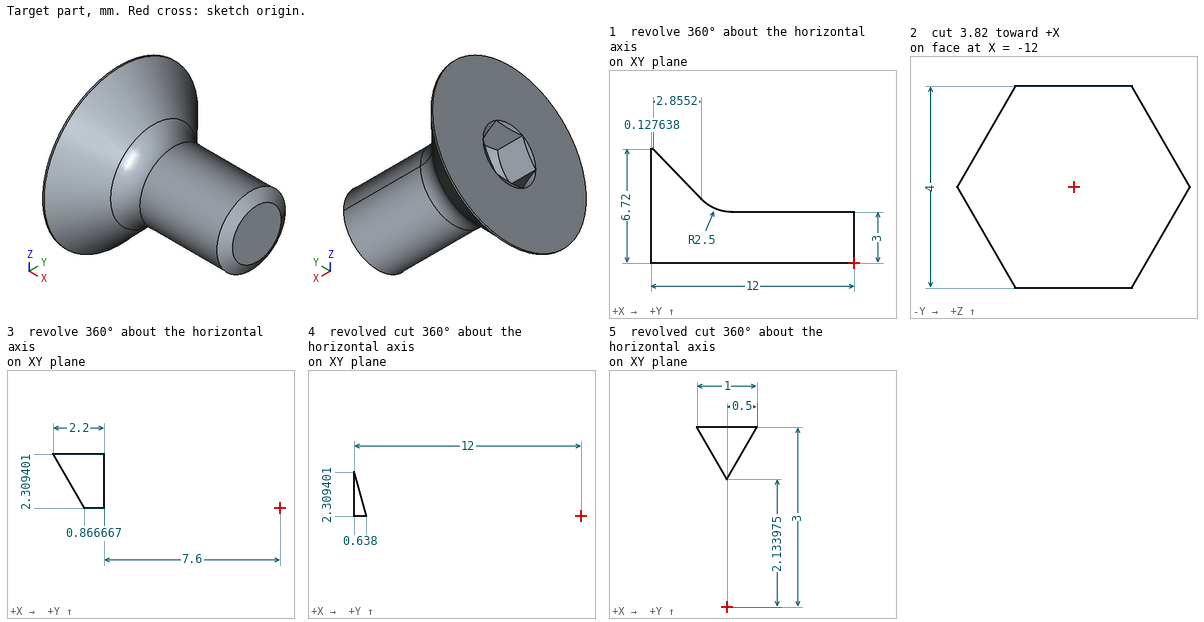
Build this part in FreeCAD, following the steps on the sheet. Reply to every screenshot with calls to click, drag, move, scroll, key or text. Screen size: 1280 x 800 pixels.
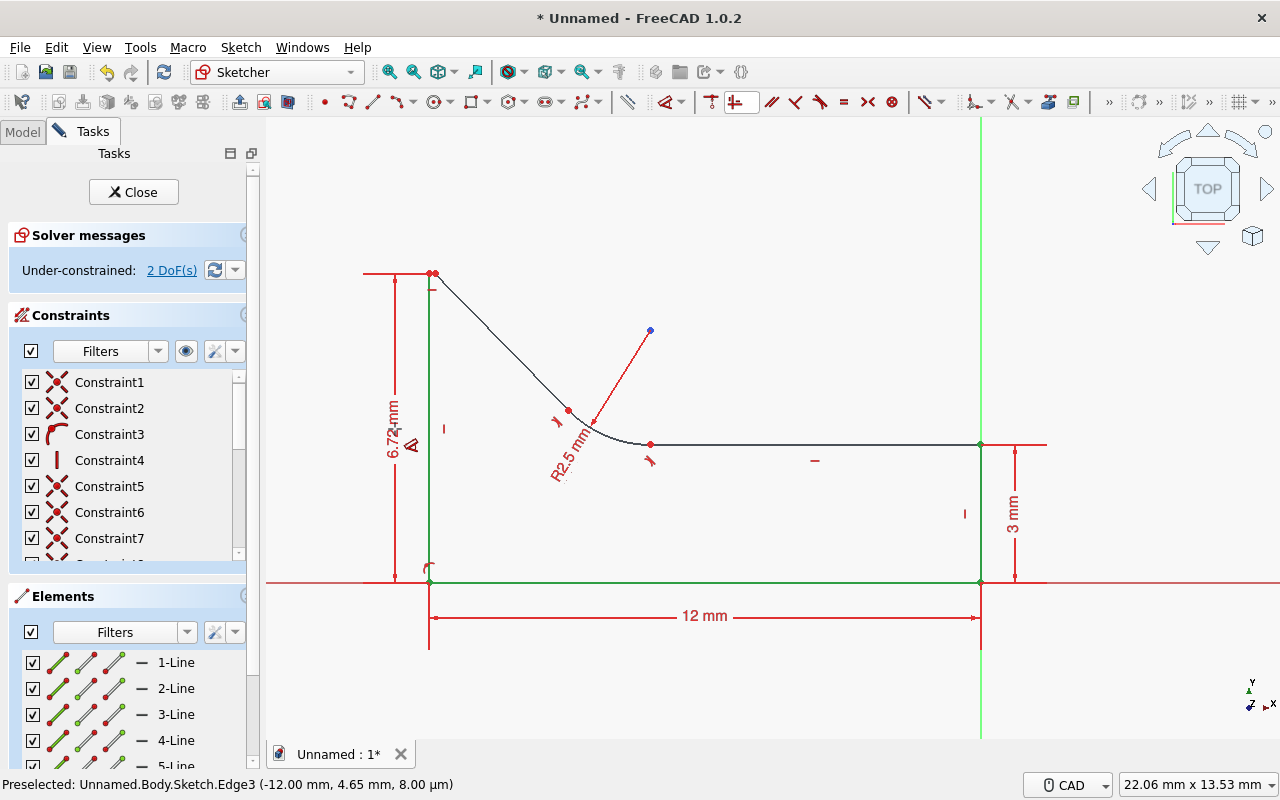
click(529, 369)
click(502, 240)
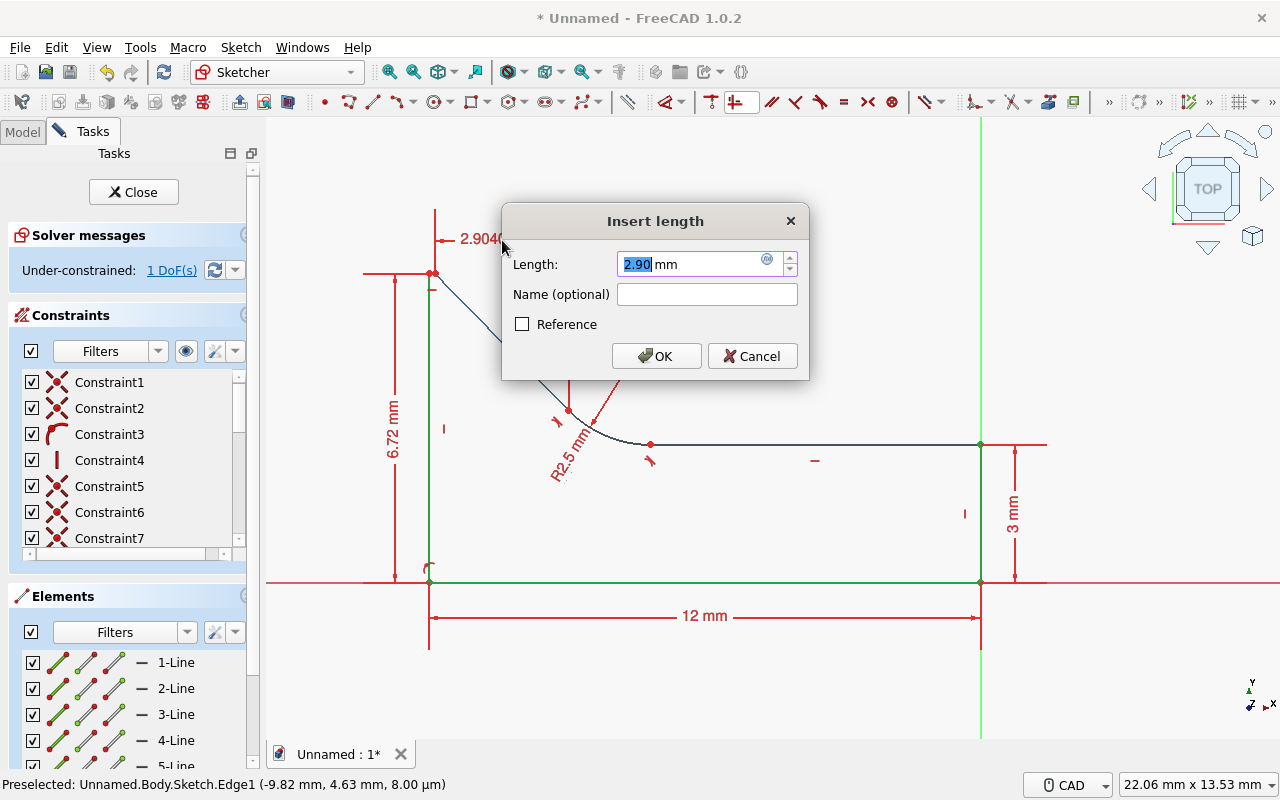
text(2.8552)
key(Return)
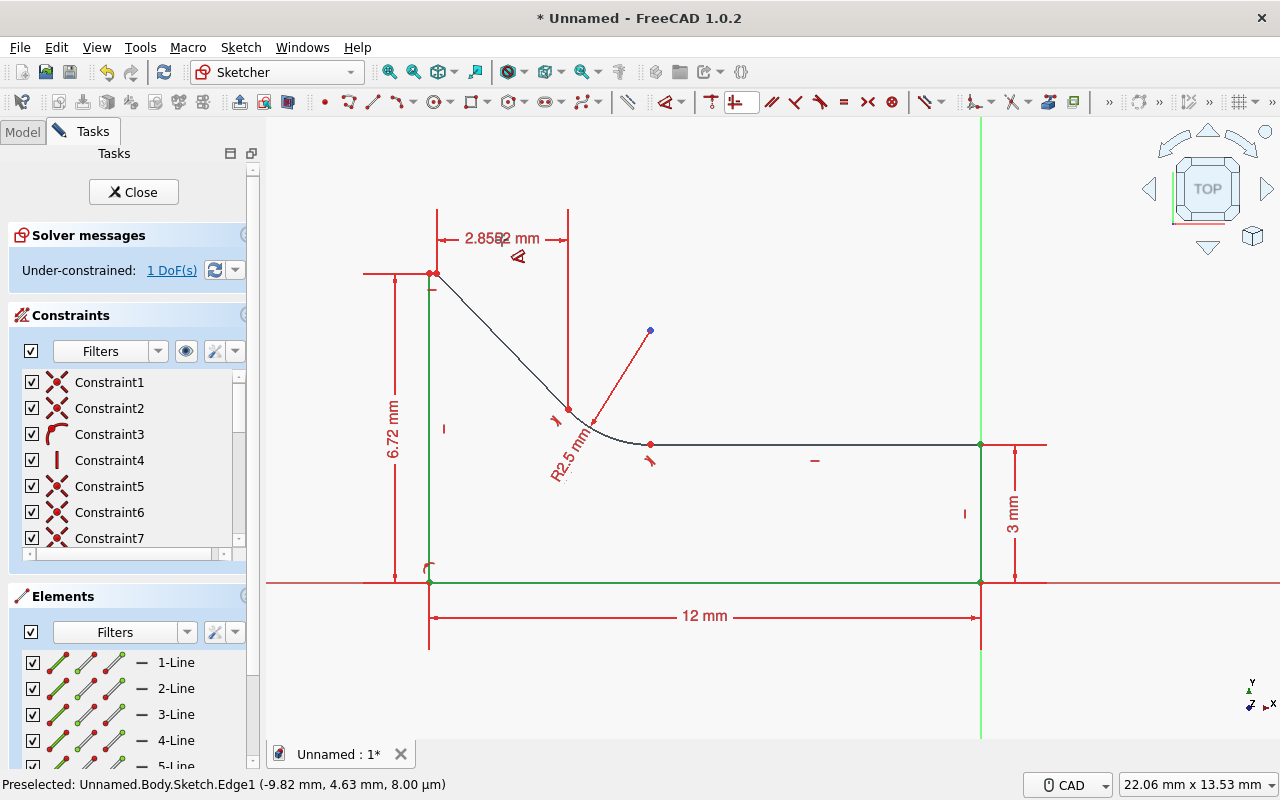
scroll(433, 274, up, 10)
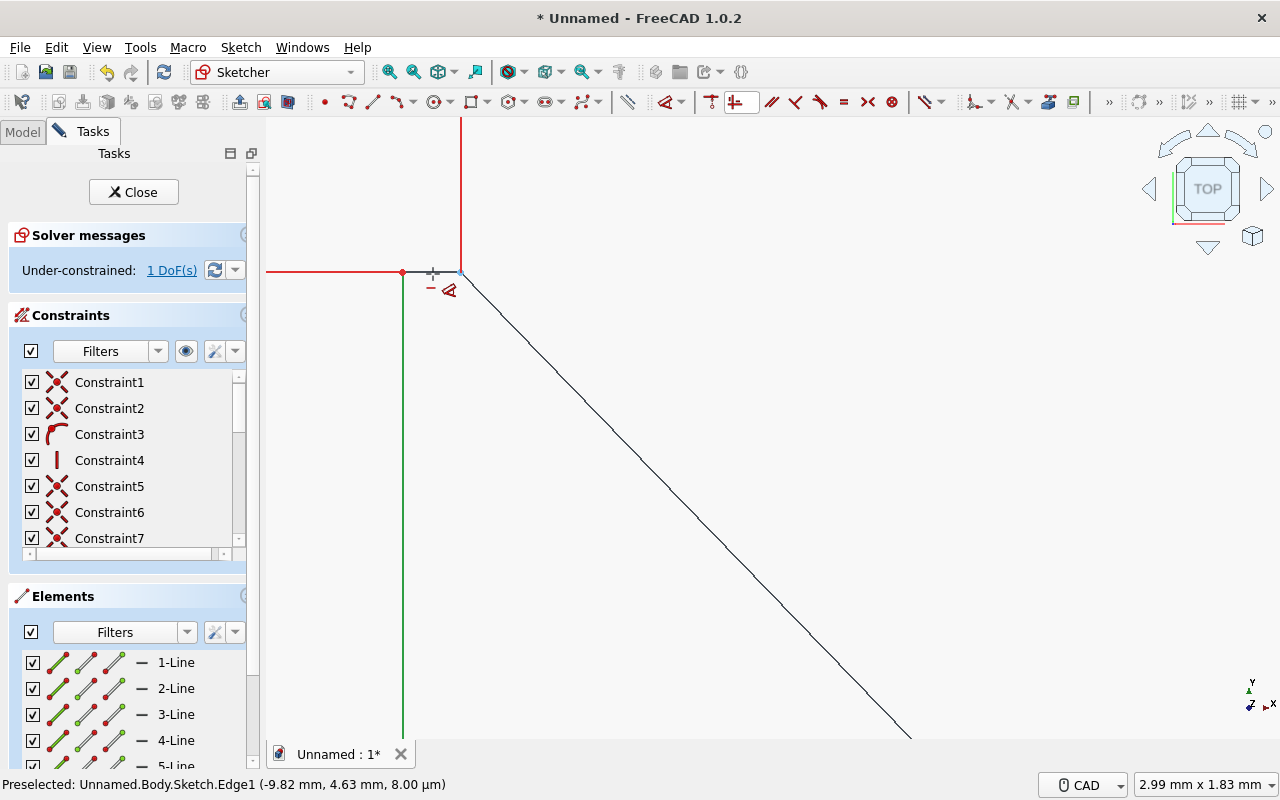
click(432, 272)
click(432, 238)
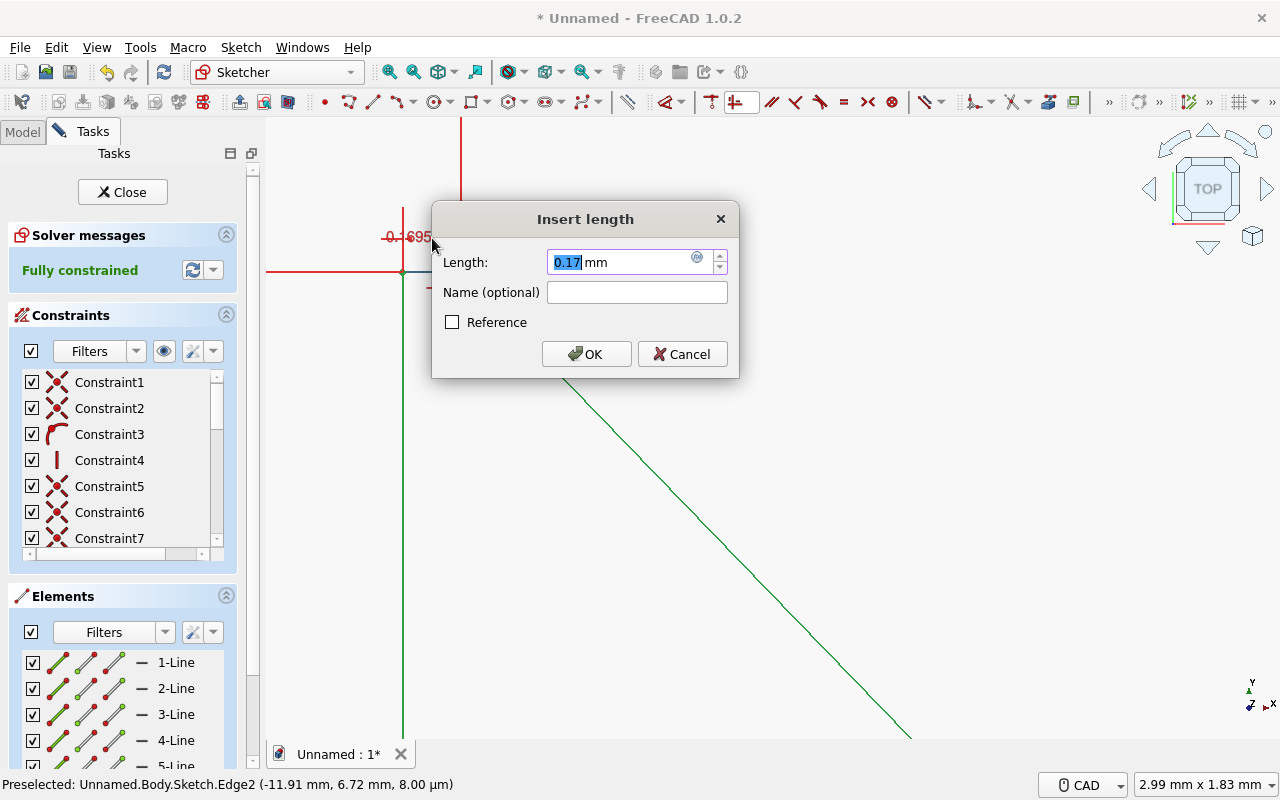
text(0.127638)
key(Return)
key(Escape)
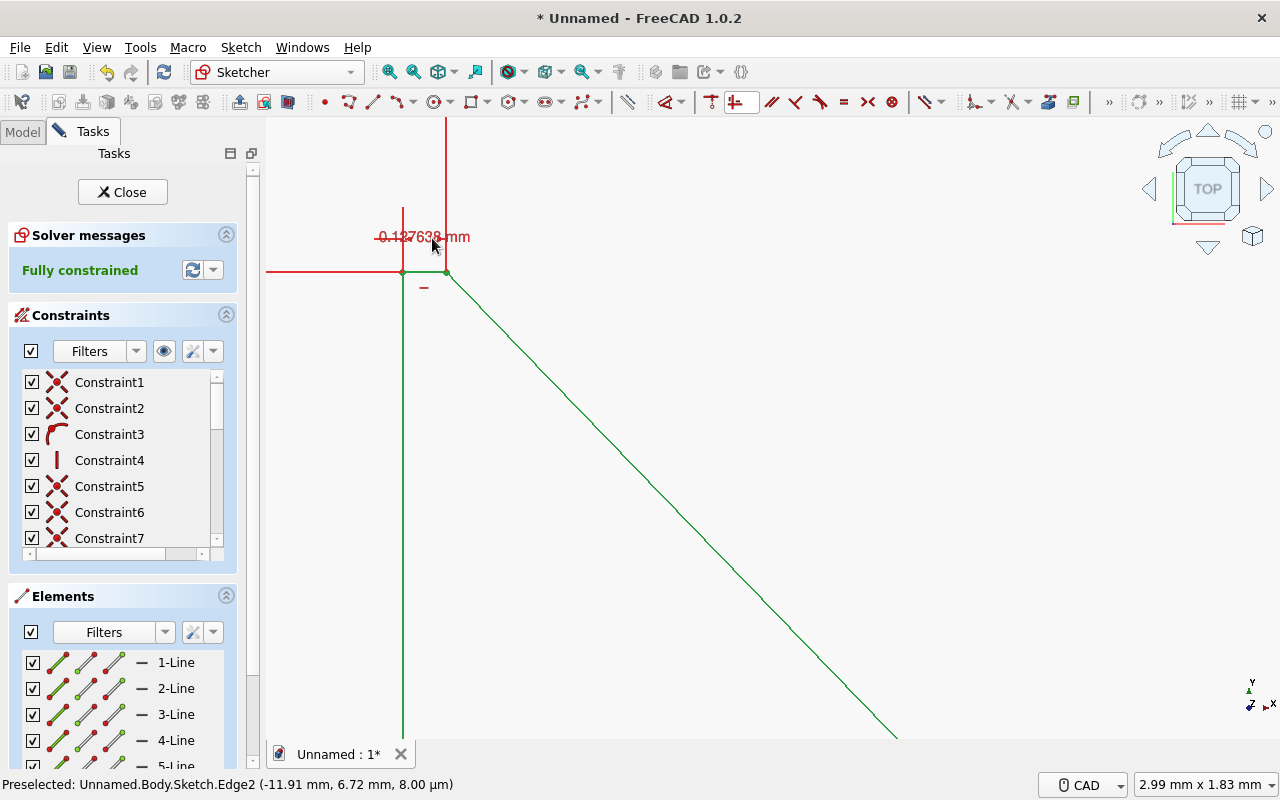
click(123, 192)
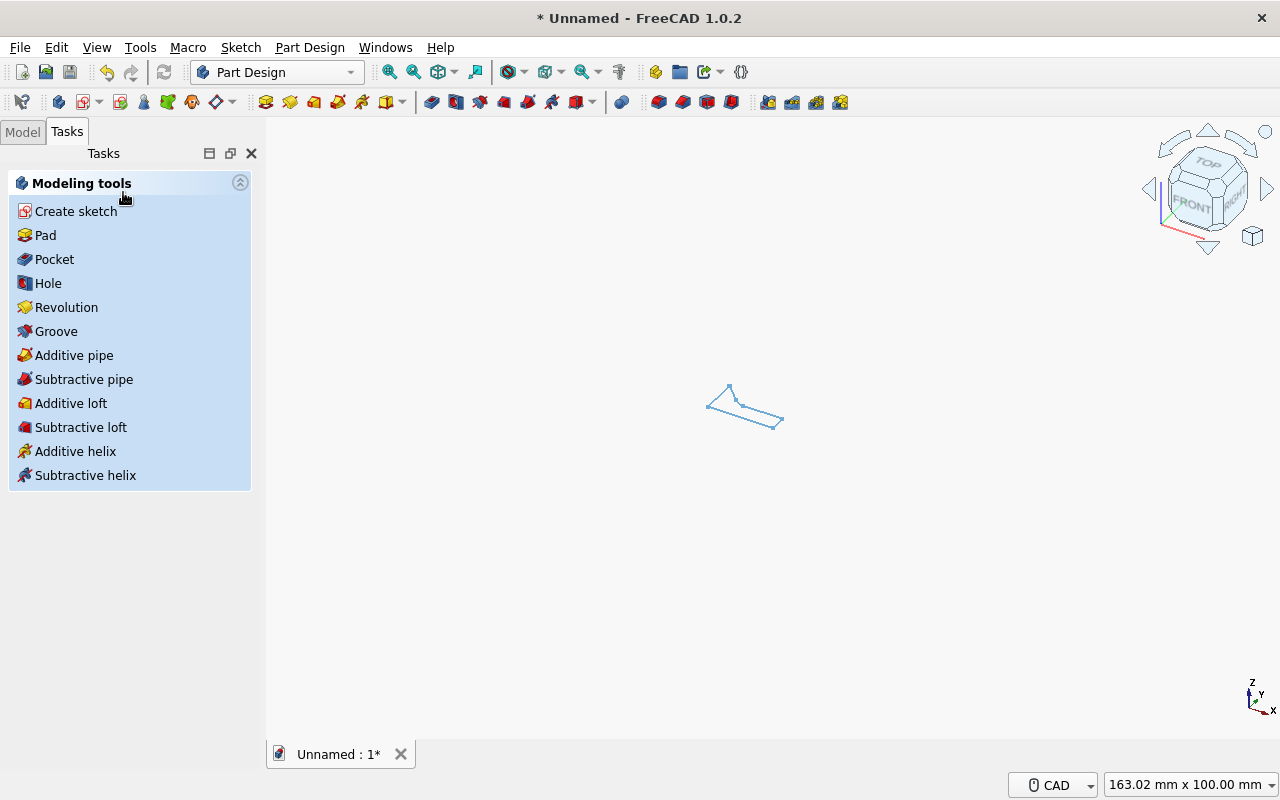
click(290, 102)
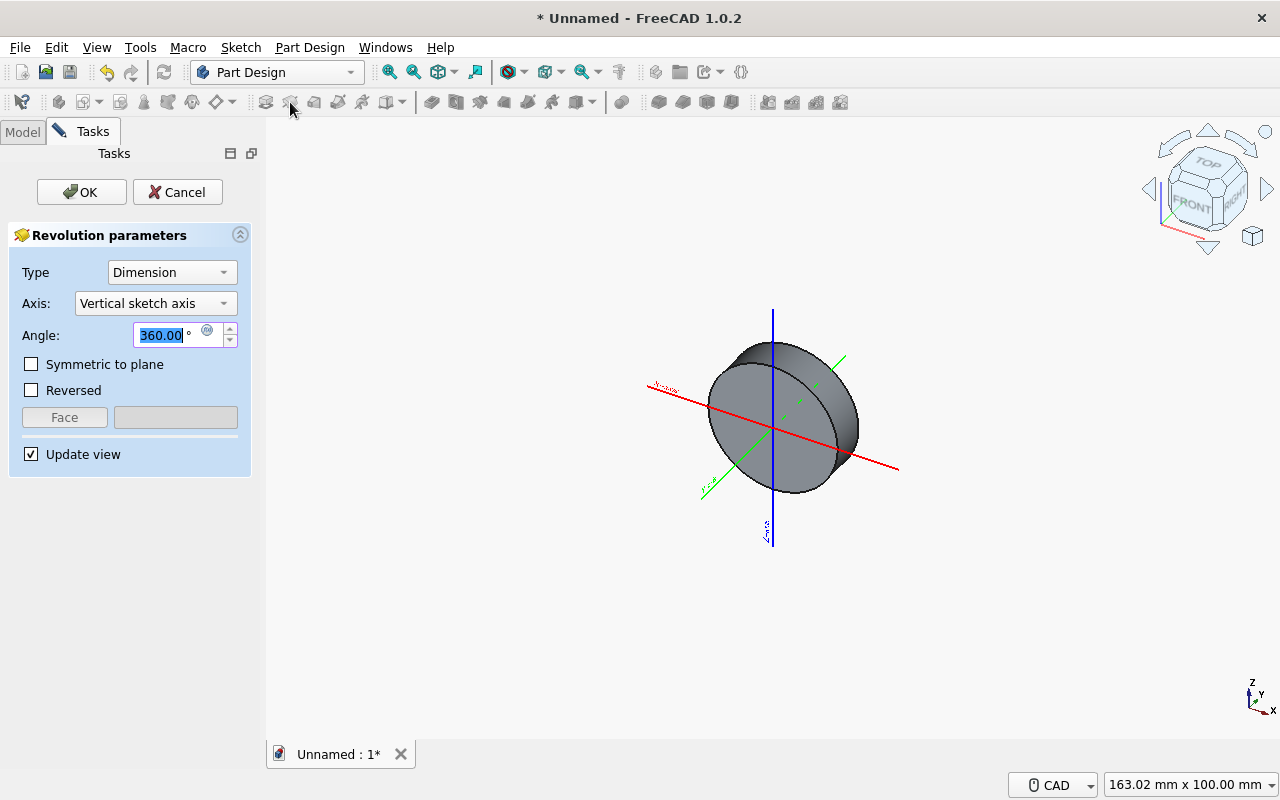
click(156, 304)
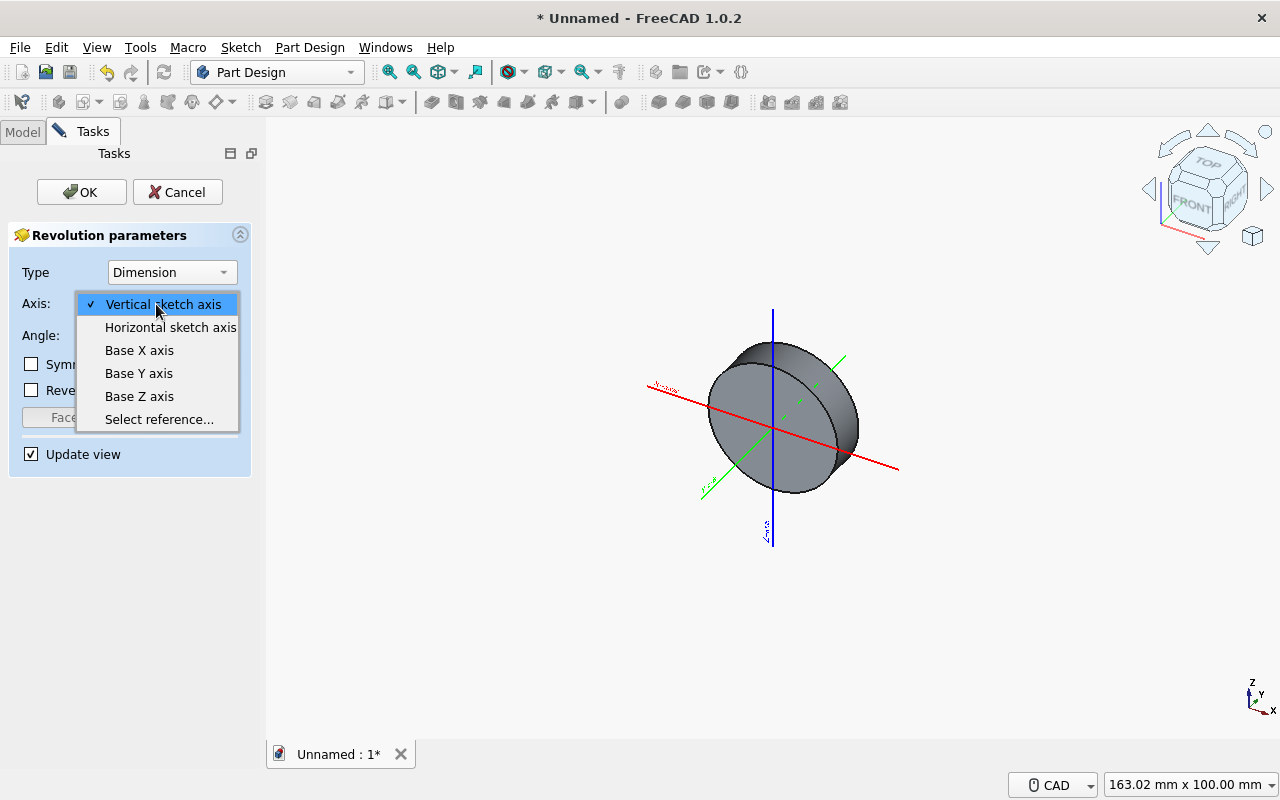
click(156, 328)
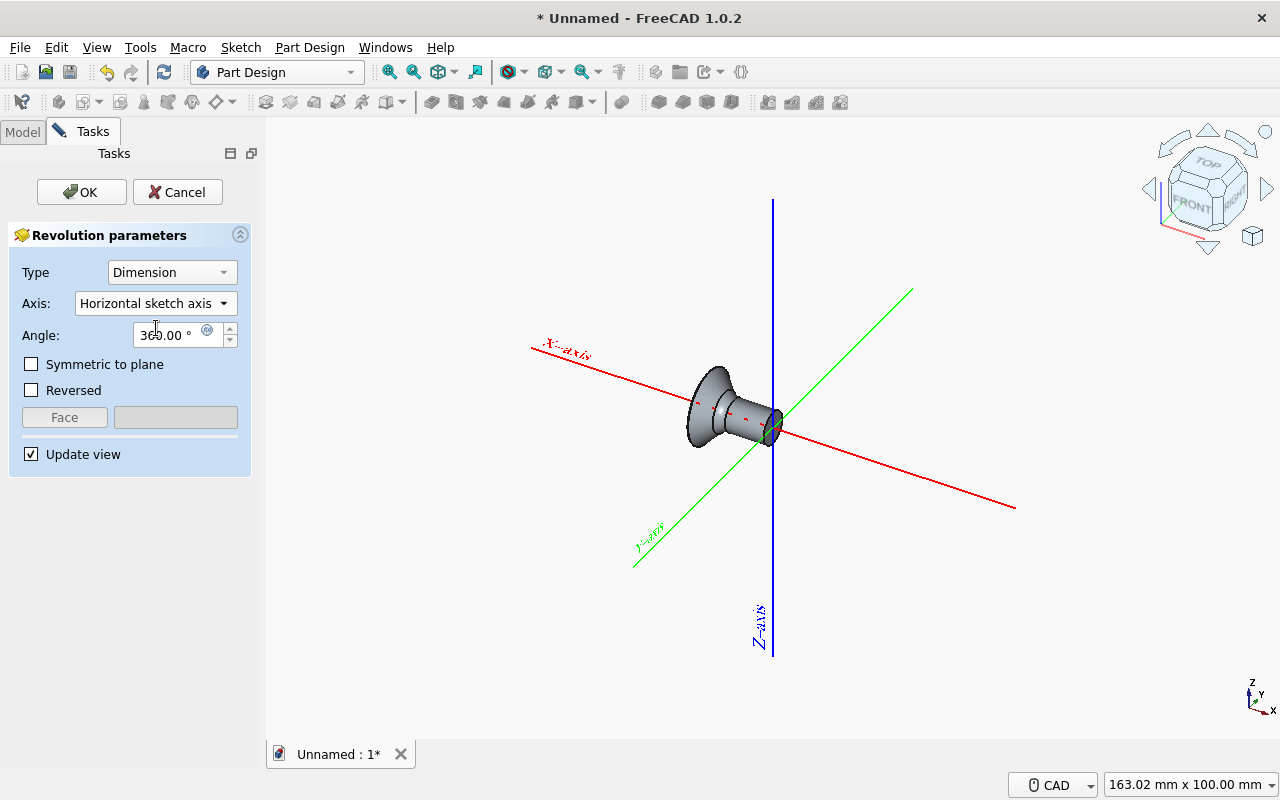
click(82, 192)